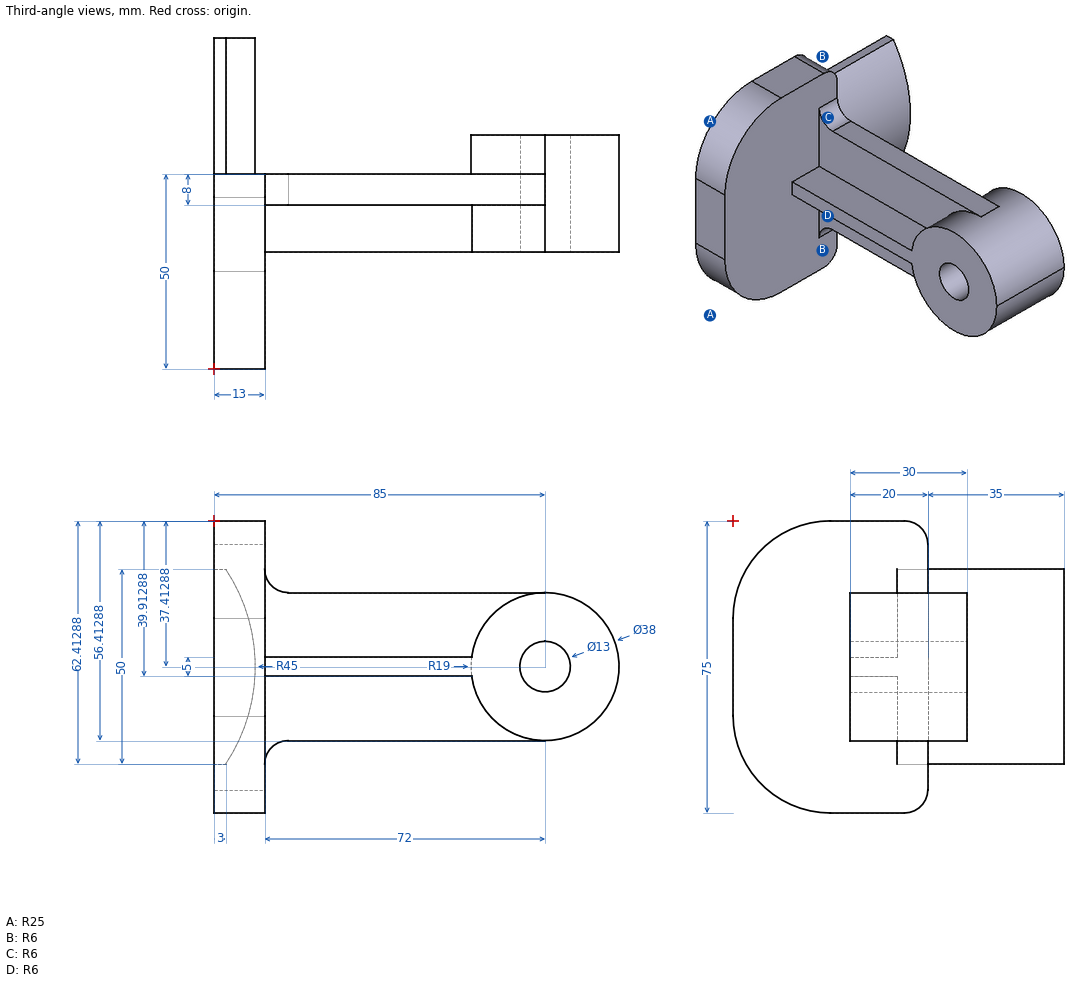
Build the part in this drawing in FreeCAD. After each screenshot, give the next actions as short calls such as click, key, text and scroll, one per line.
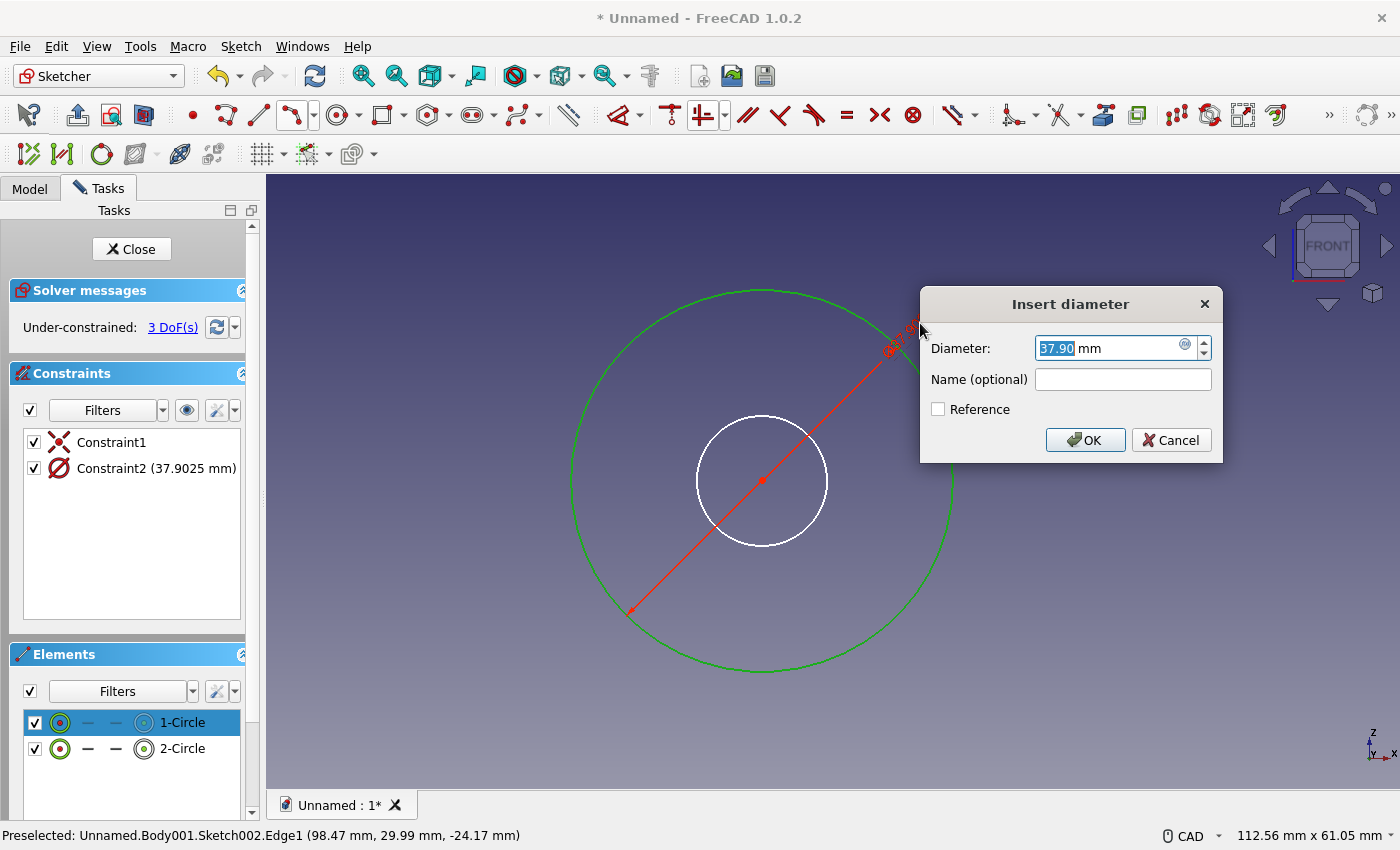
text(38)
key(Return)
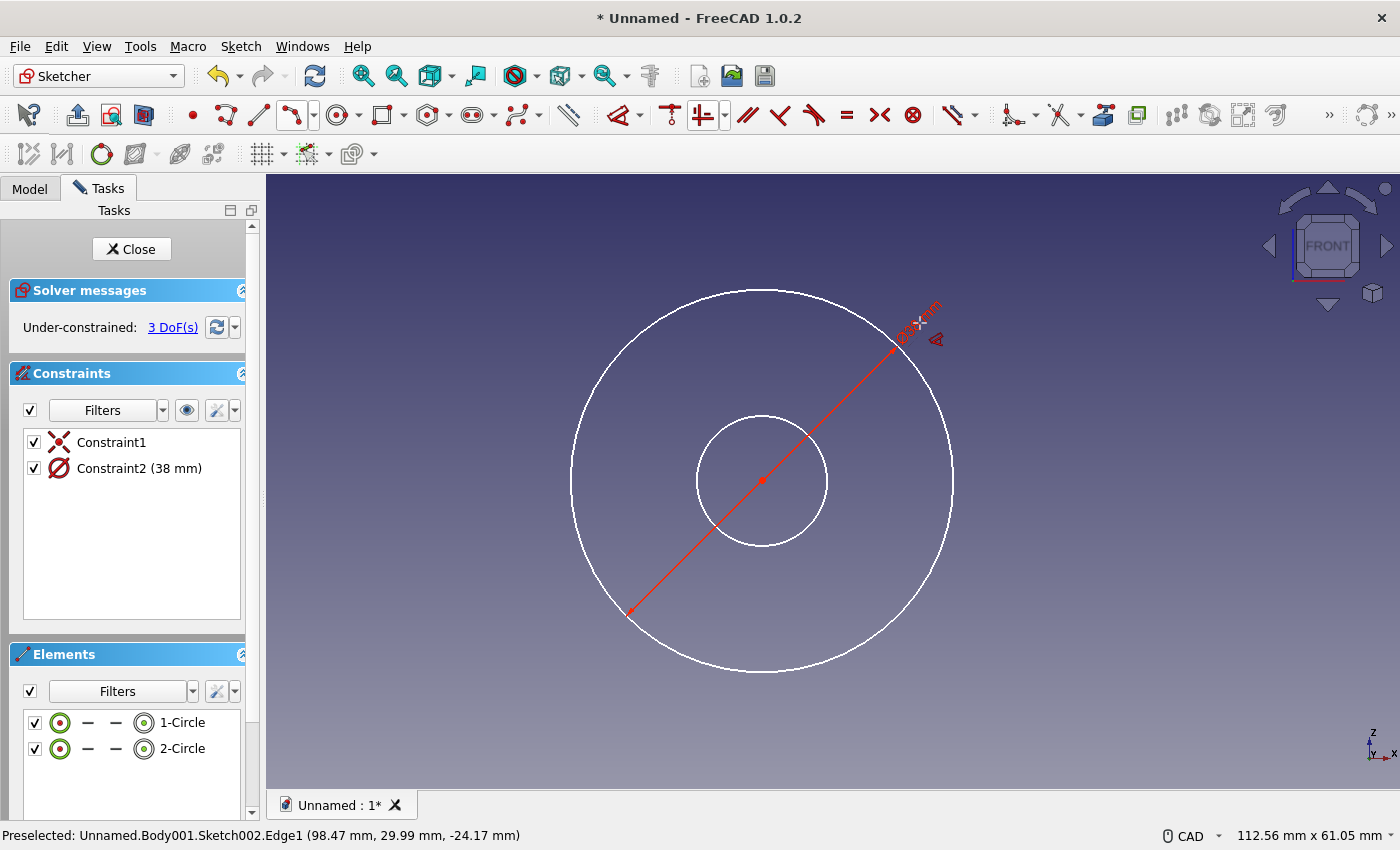
click(808, 435)
click(831, 412)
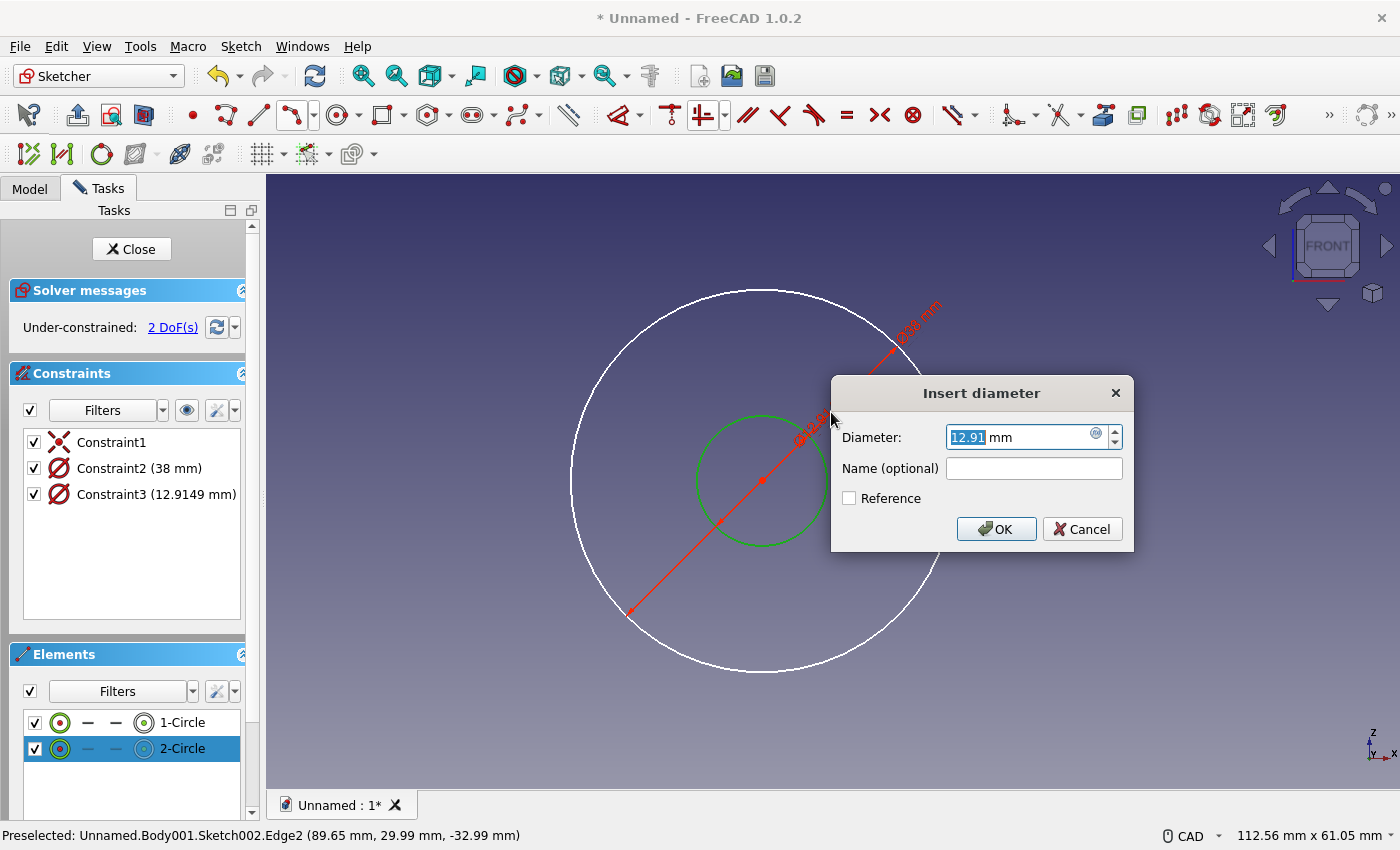
text(13)
key(Return)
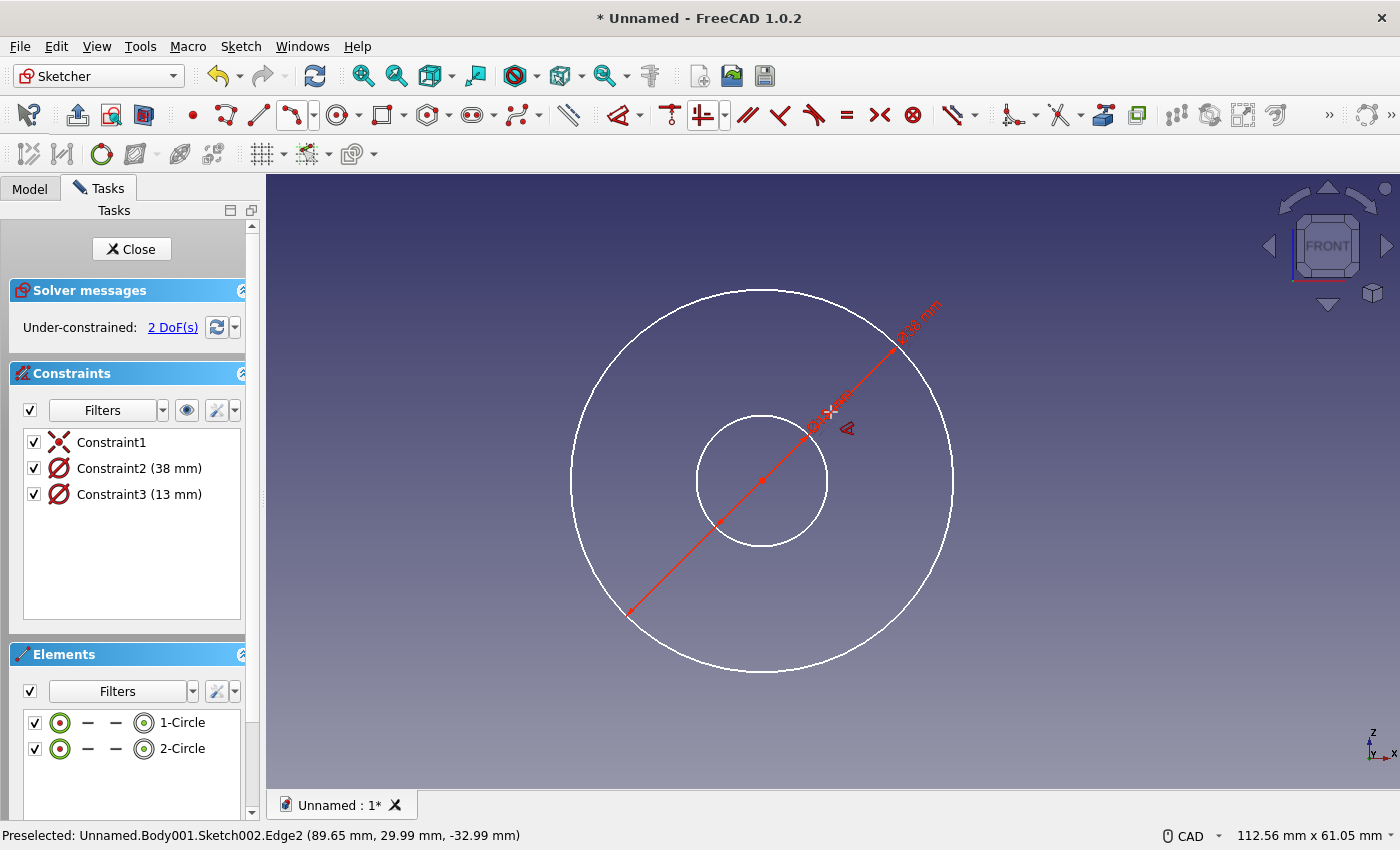
click(762, 481)
click(528, 515)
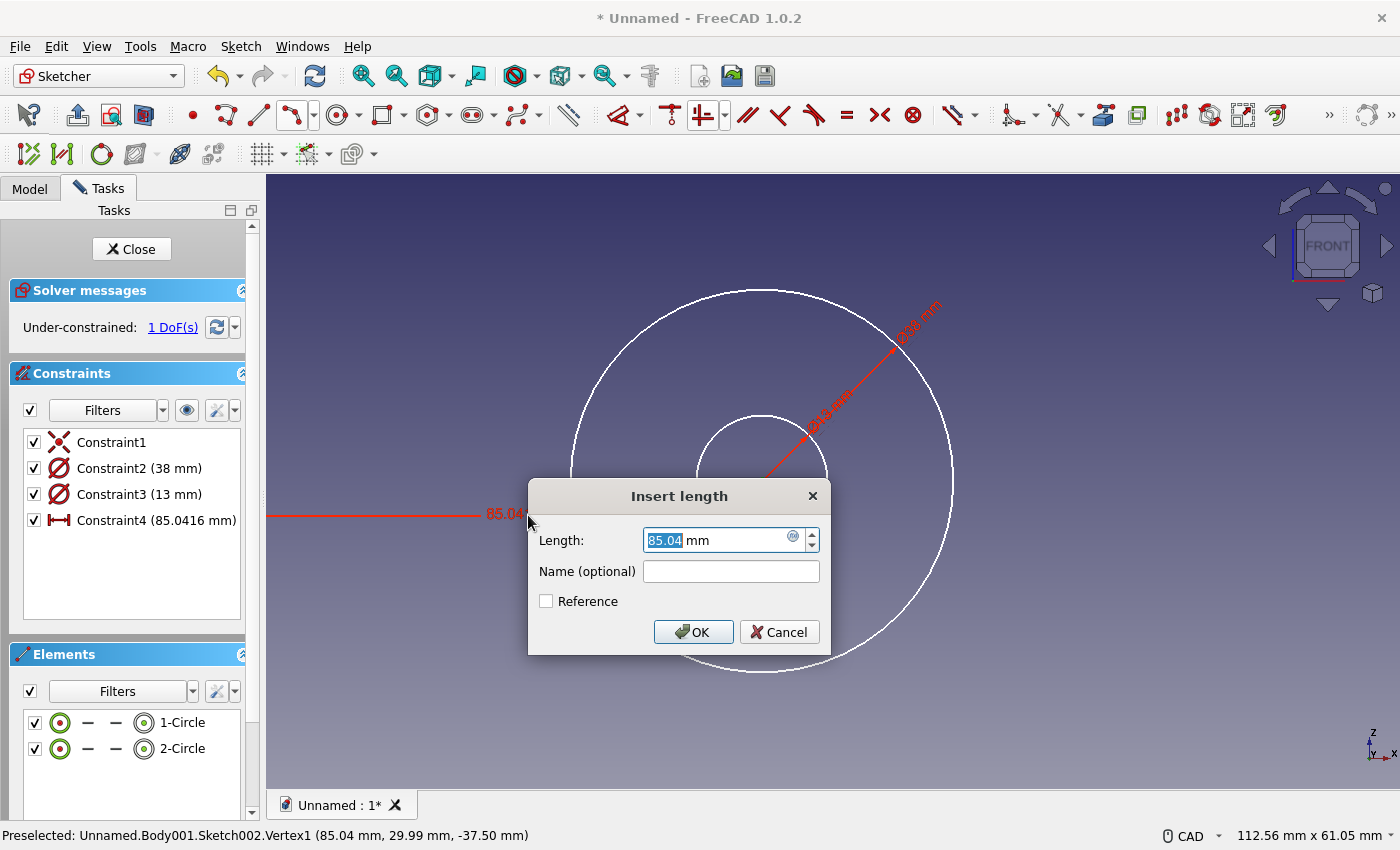
text(85)
key(Return)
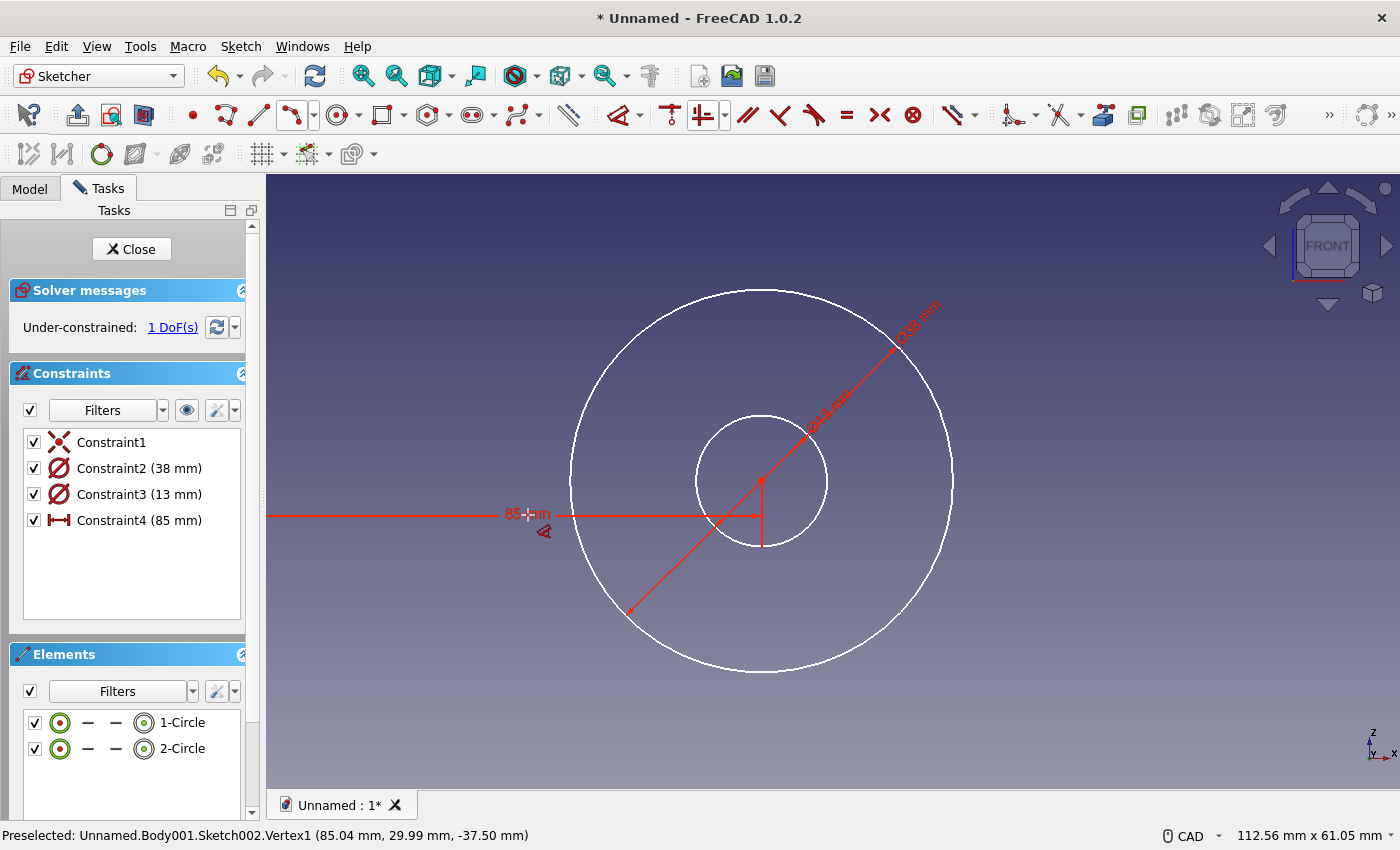
click(762, 481)
click(796, 341)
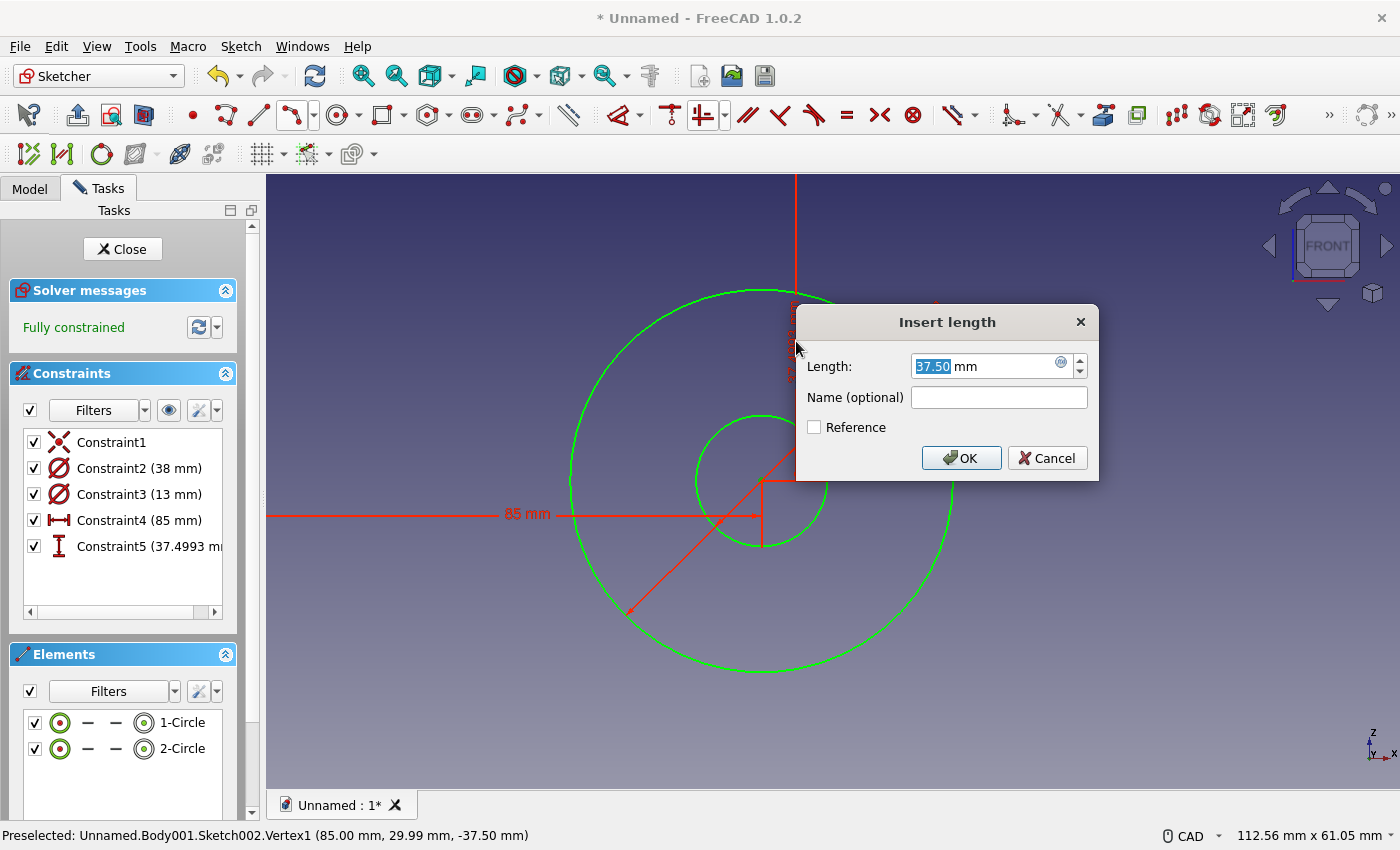
text(37.41288)
key(Return)
key(Escape)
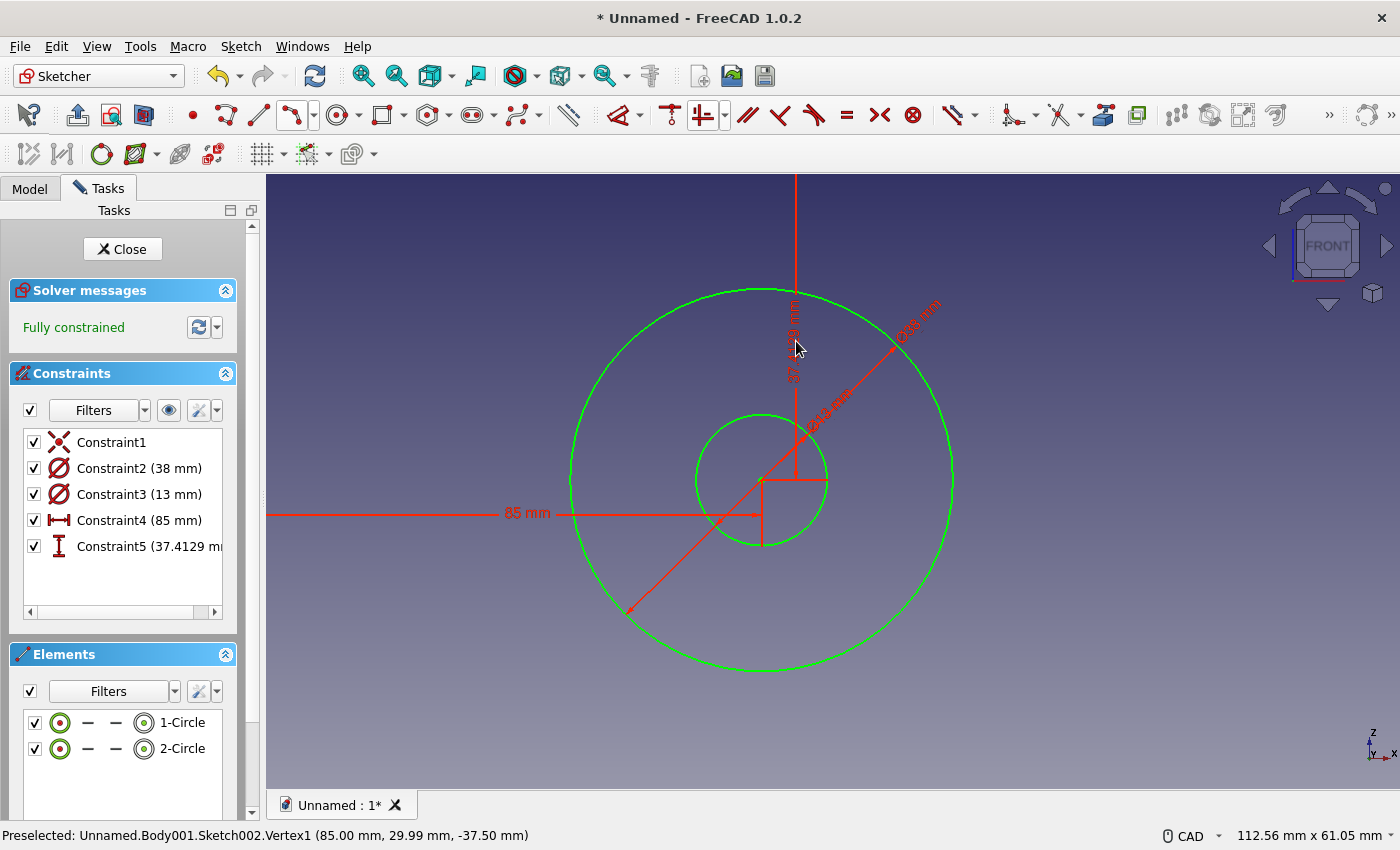
click(123, 249)